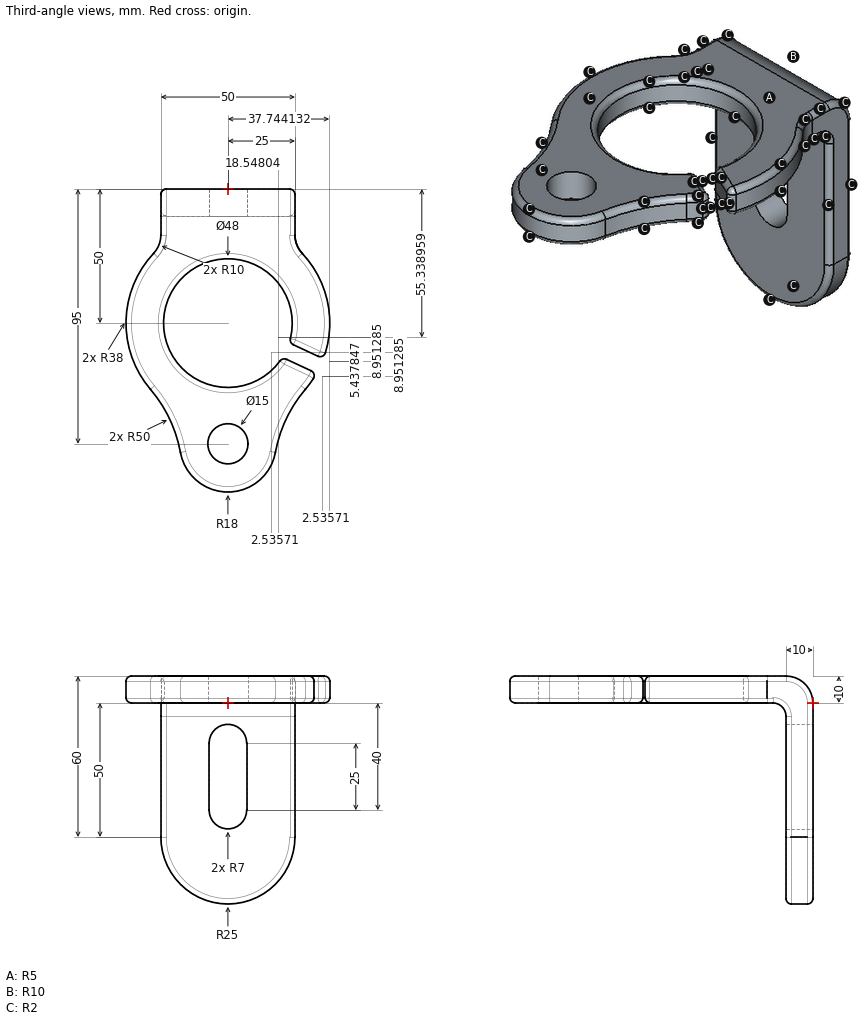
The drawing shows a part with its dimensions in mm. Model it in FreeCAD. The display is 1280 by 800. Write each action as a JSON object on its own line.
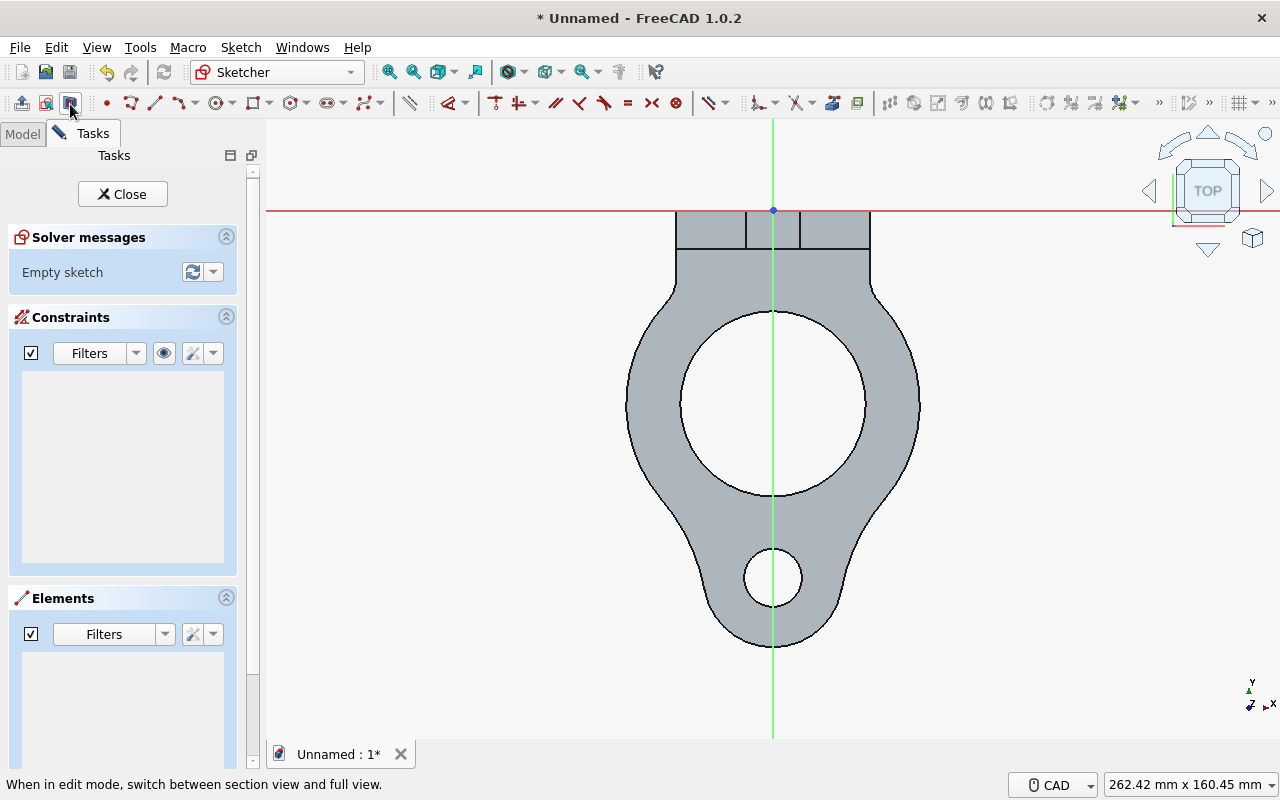
{"action": "scroll", "coordinate": [904, 456], "scroll_direction": "up", "scroll_amount": 10}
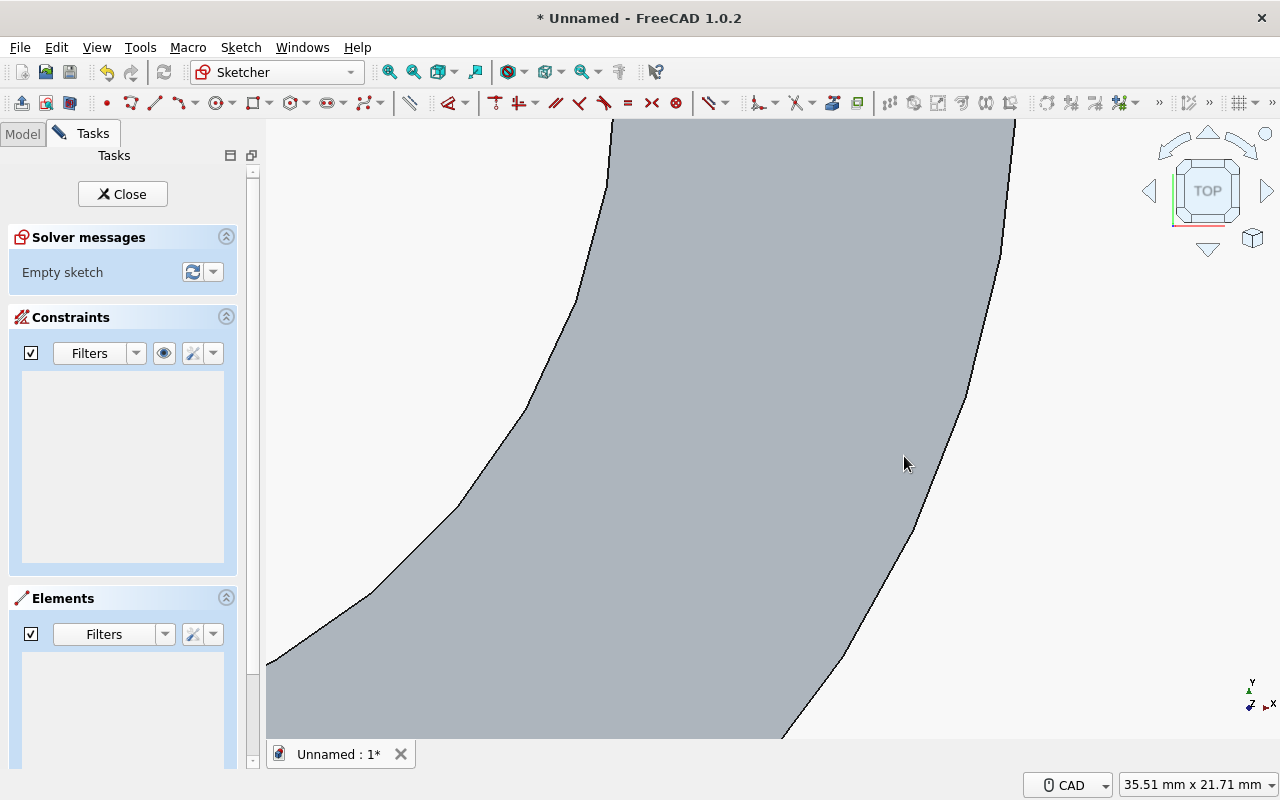
{"action": "left_click", "coordinate": [132, 104]}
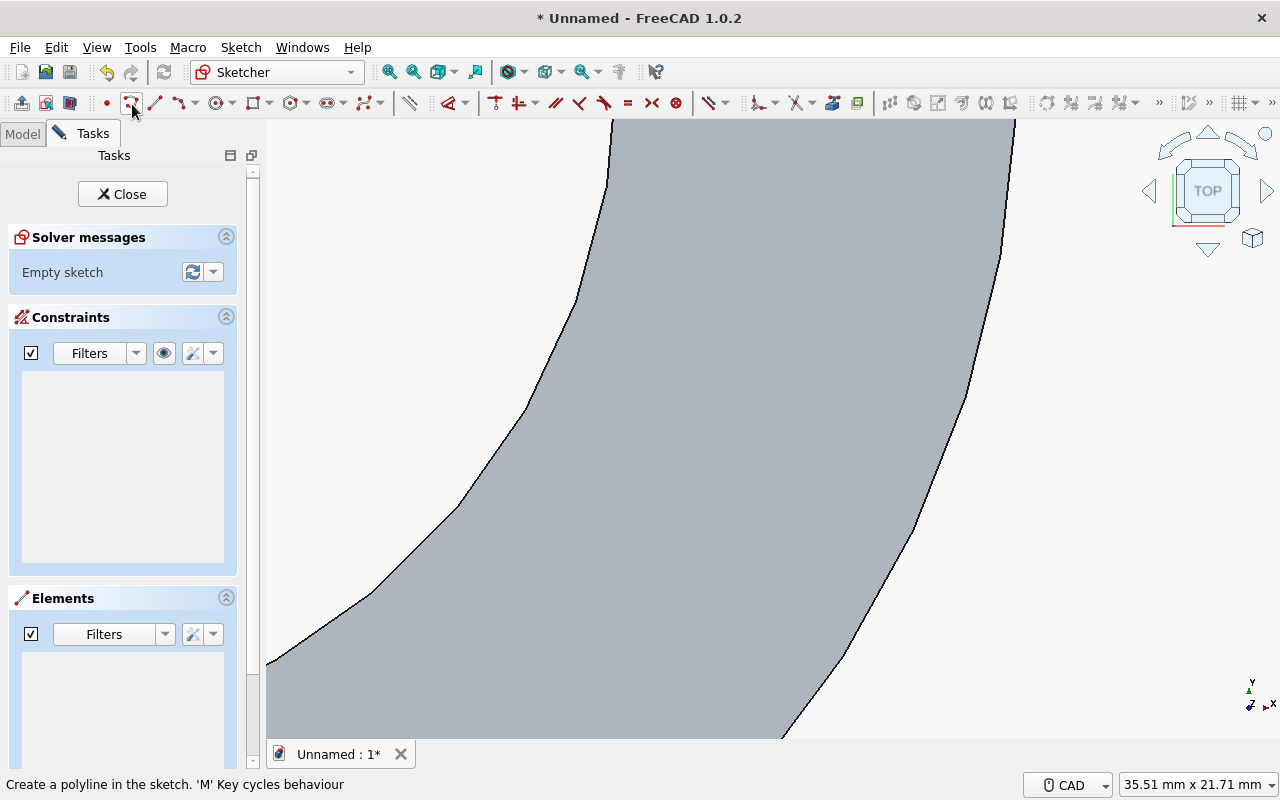
{"action": "left_click", "coordinate": [462, 220]}
{"action": "left_click", "coordinate": [1010, 475]}
{"action": "left_click", "coordinate": [937, 631]}
{"action": "left_click", "coordinate": [389, 375]}
{"action": "left_click", "coordinate": [462, 221]}
{"action": "key", "text": "Escape"}
{"action": "key", "text": "Escape"}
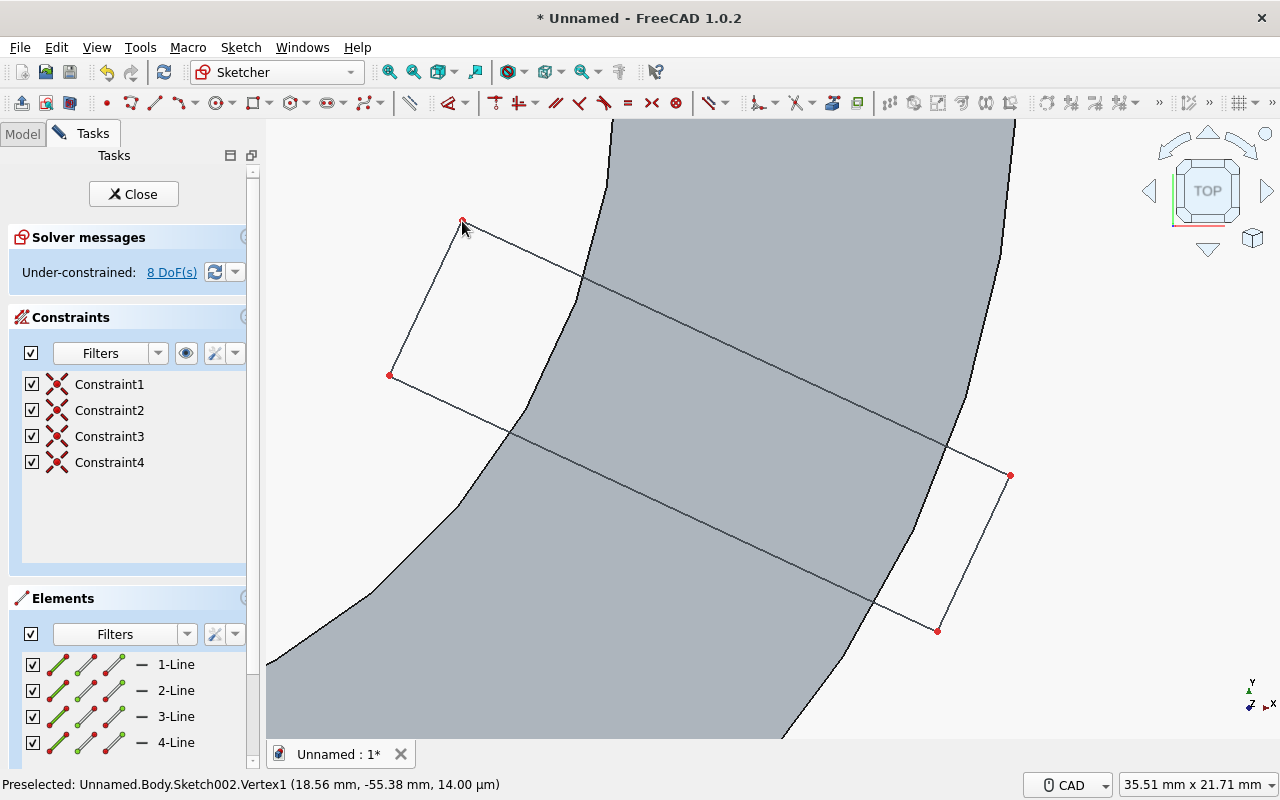
{"action": "left_click", "coordinate": [448, 104]}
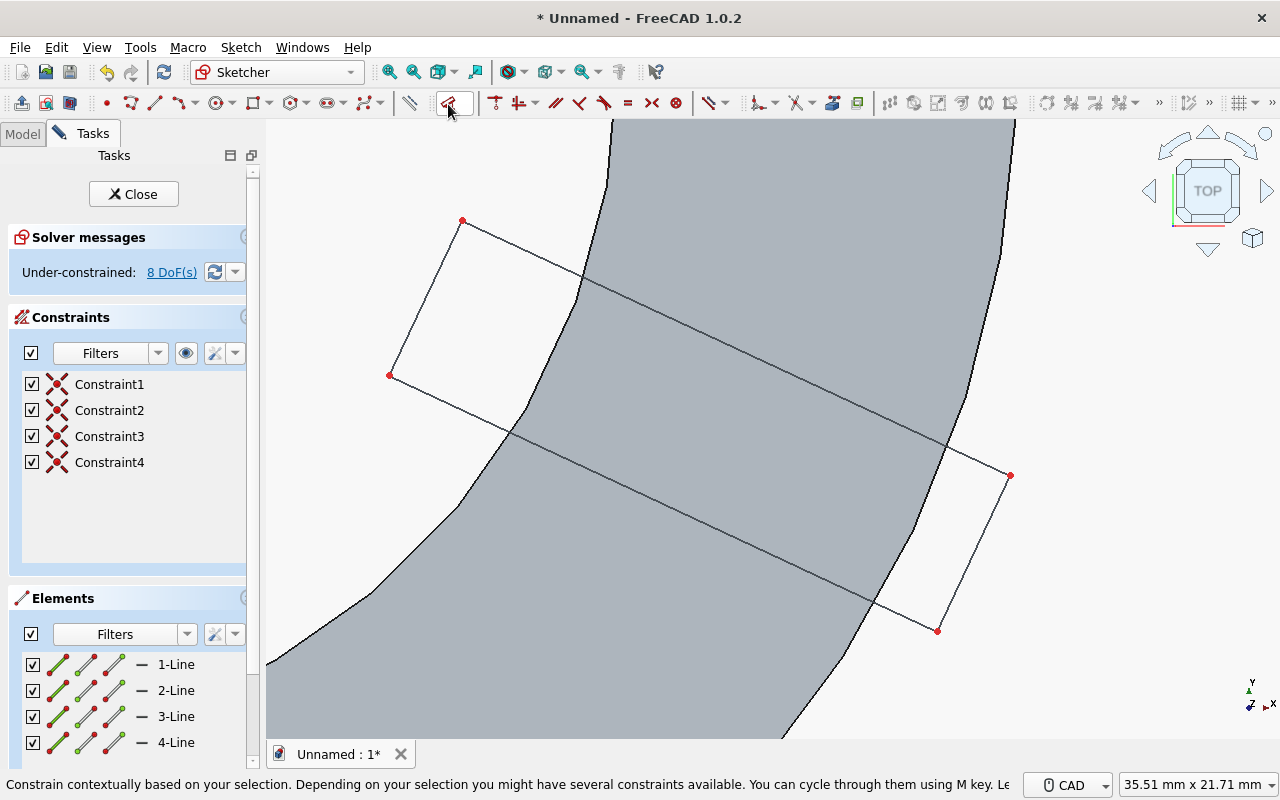
{"action": "left_click", "coordinate": [988, 523]}
{"action": "left_click", "coordinate": [974, 666]}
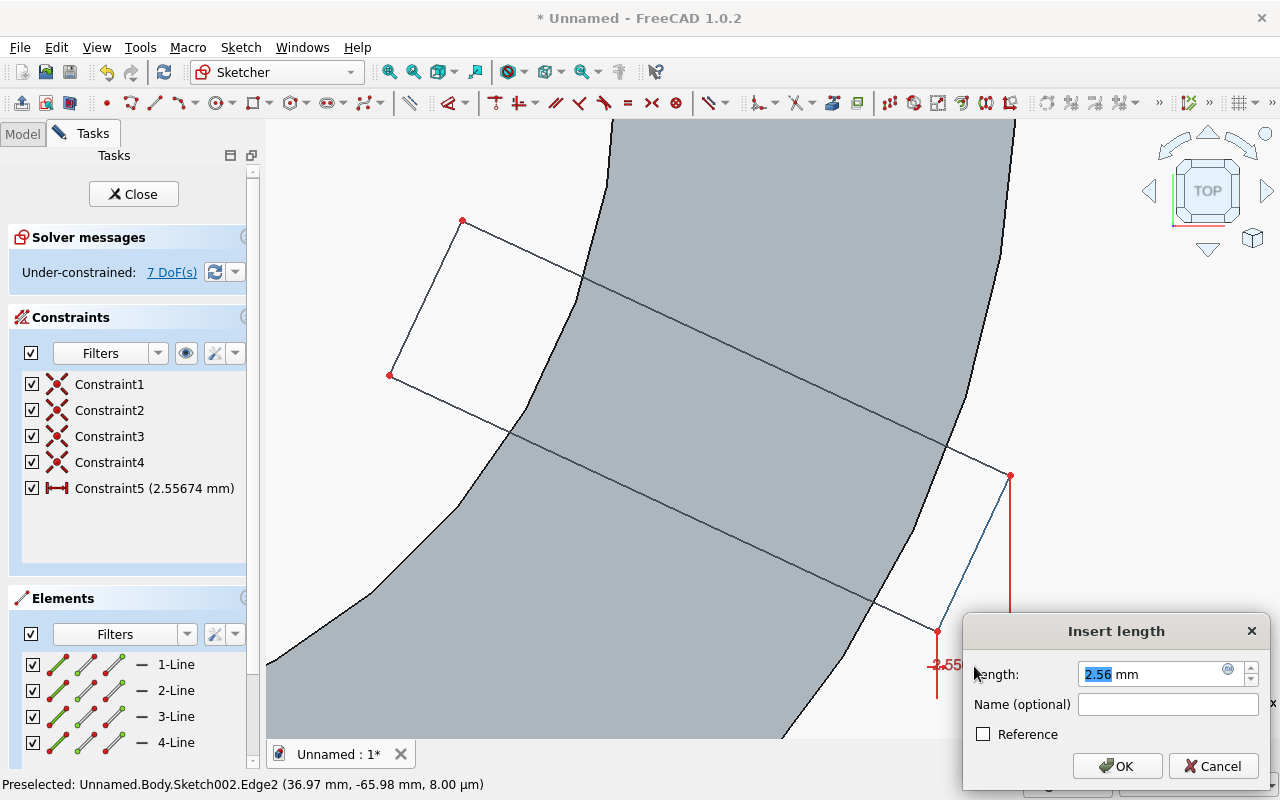
{"action": "type", "text": "2.53571"}
{"action": "key", "text": "Return"}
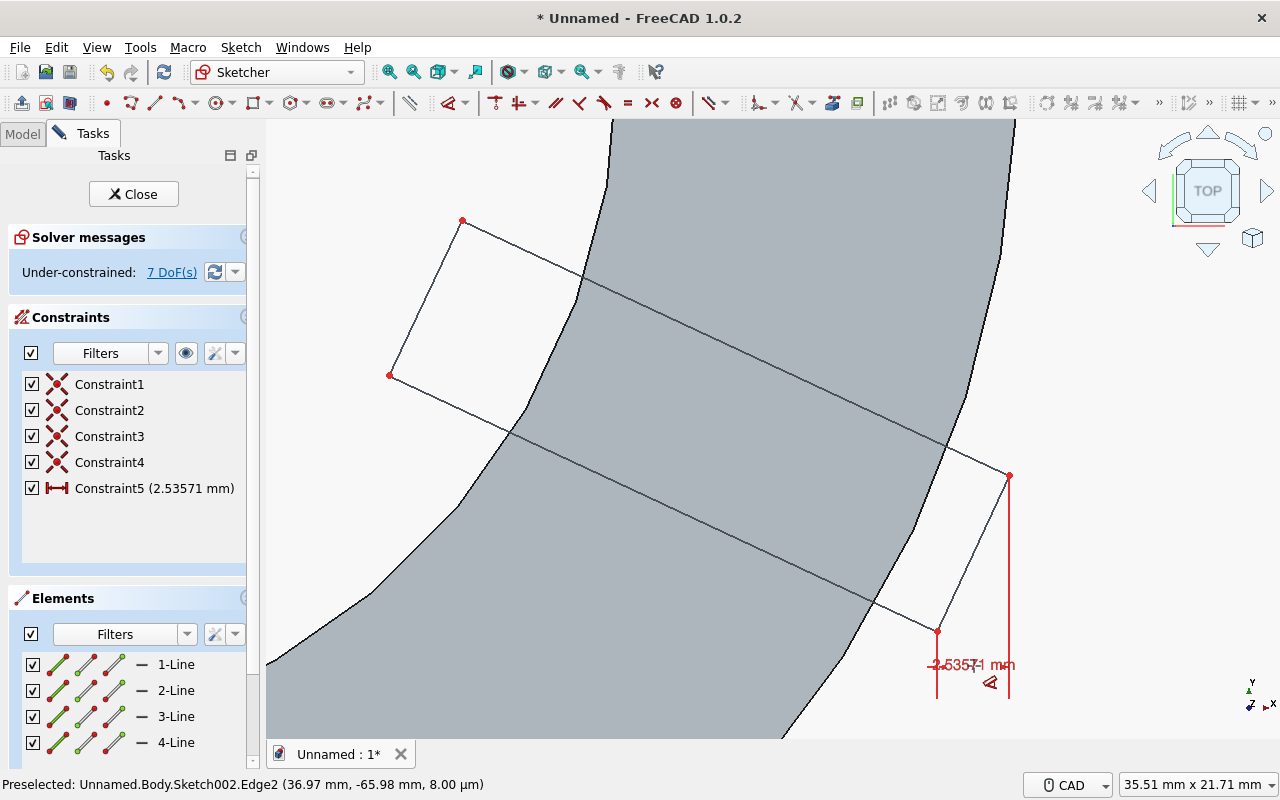
{"action": "left_click", "coordinate": [411, 330]}
{"action": "left_click", "coordinate": [425, 187]}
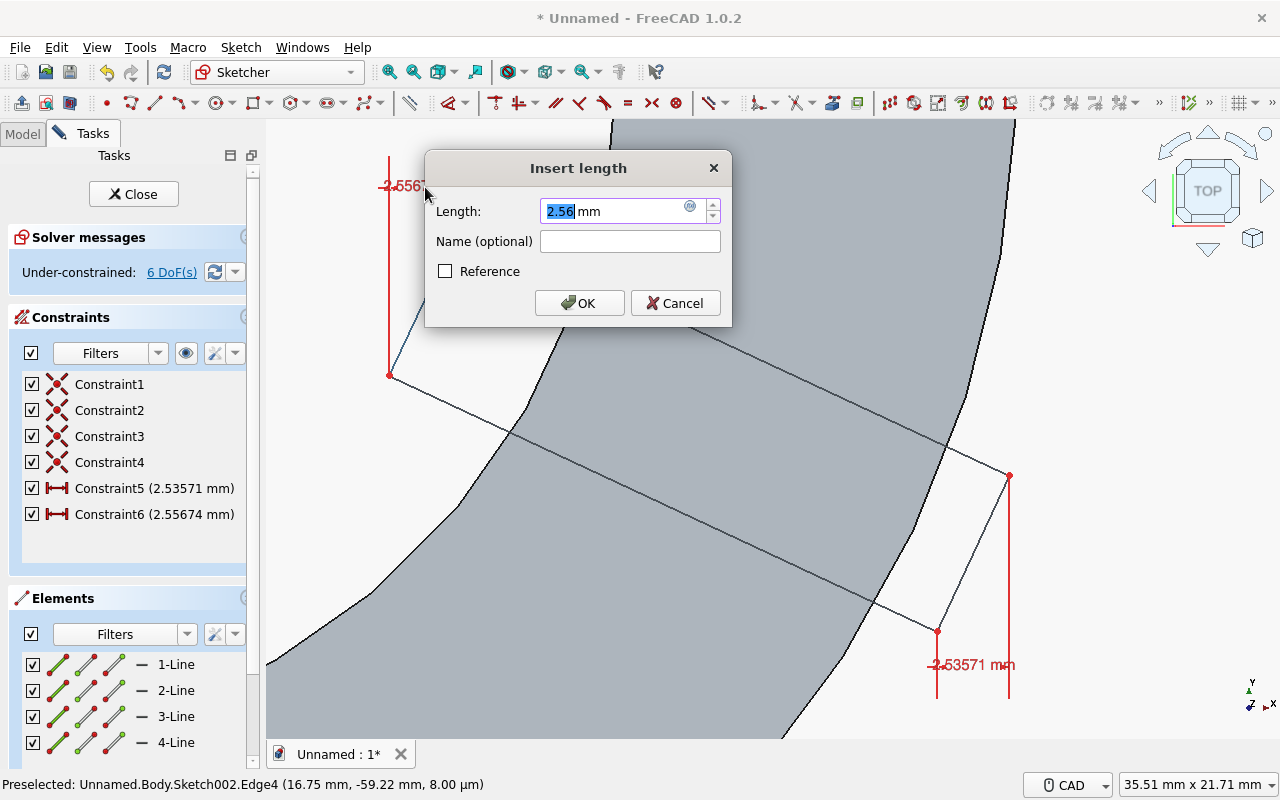
{"action": "type", "text": "2.53571"}
{"action": "key", "text": "Return"}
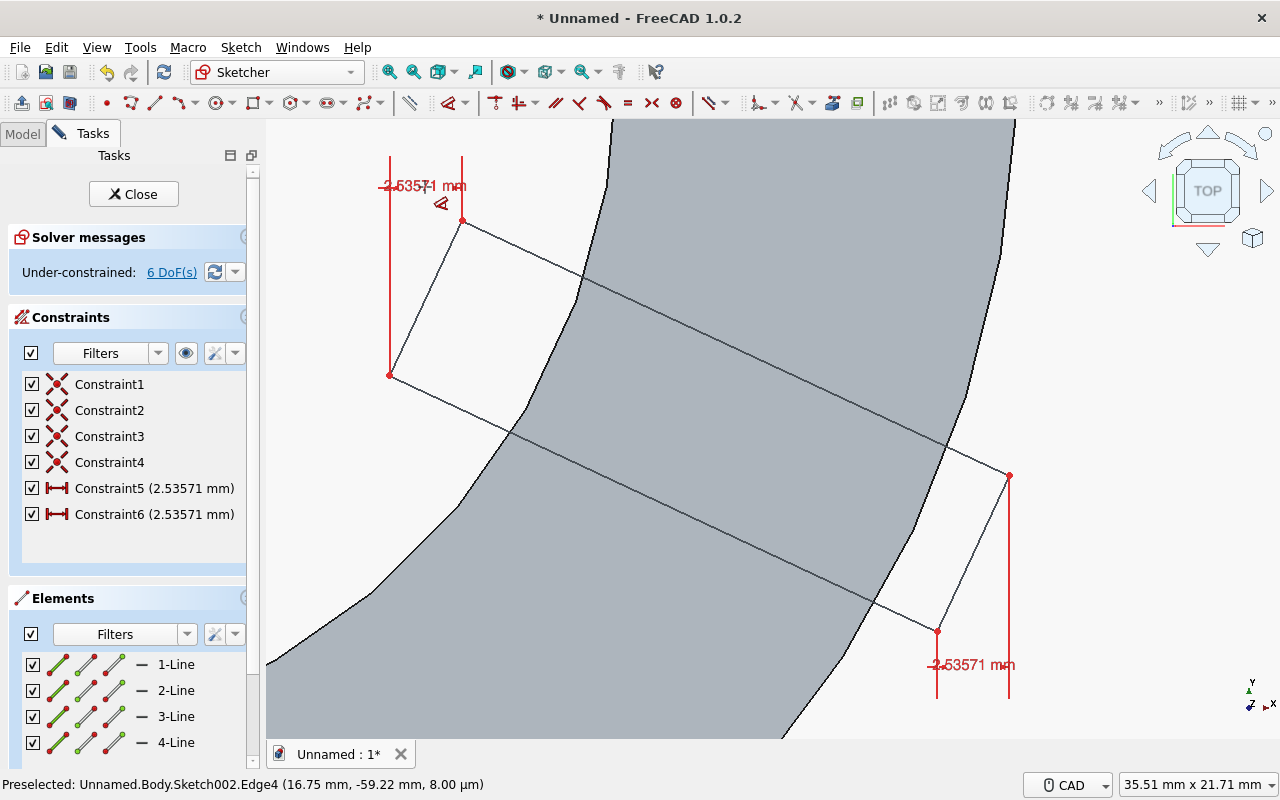
{"action": "left_click", "coordinate": [462, 221]}
{"action": "left_click", "coordinate": [378, 255]}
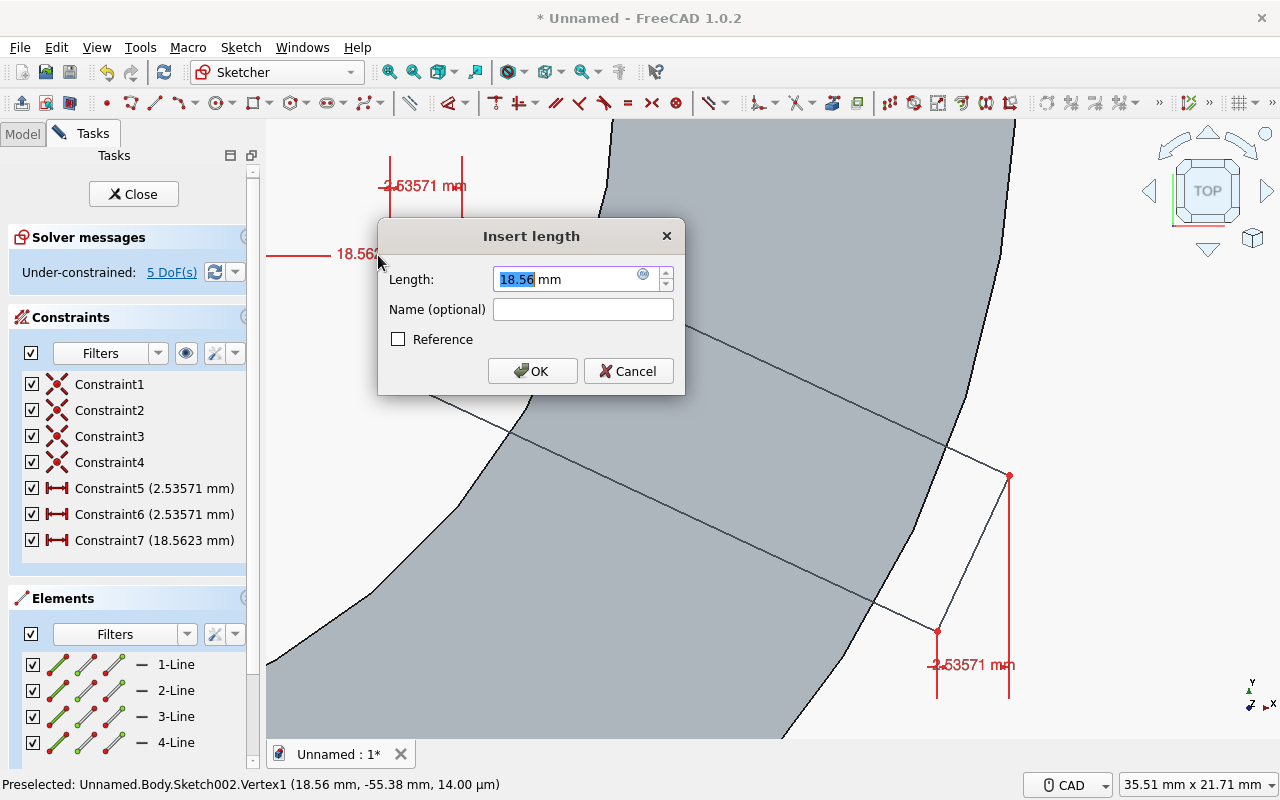
{"action": "type", "text": "18.54804"}
{"action": "key", "text": "Return"}